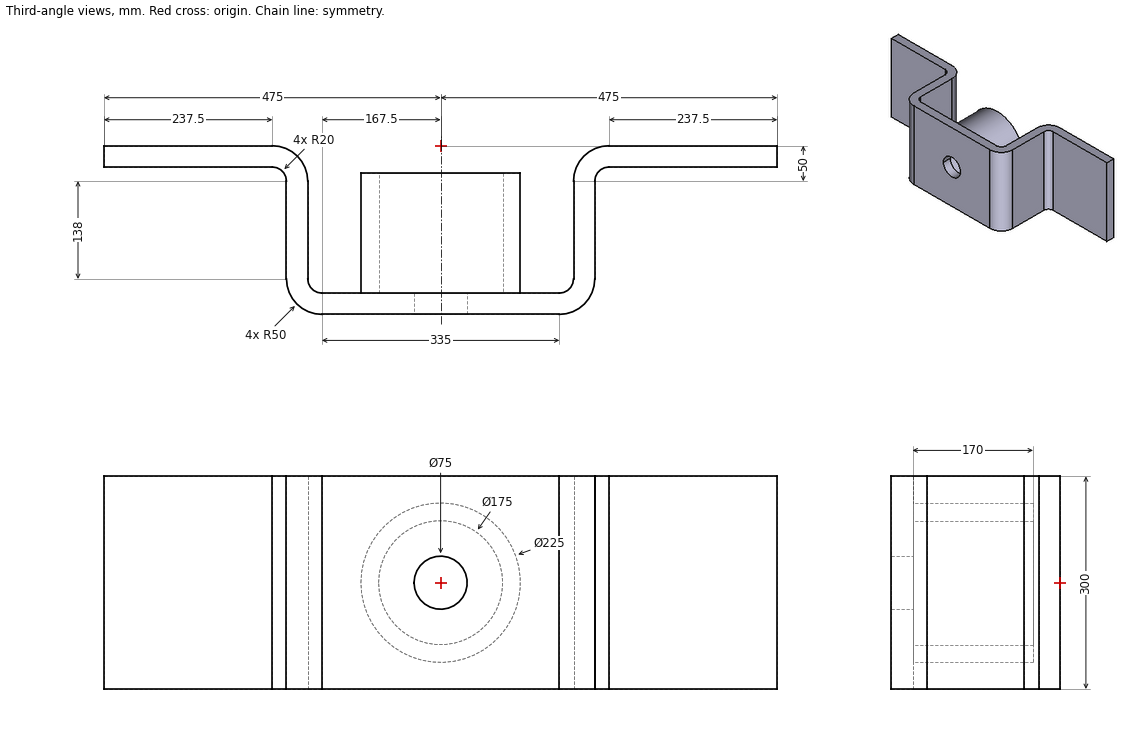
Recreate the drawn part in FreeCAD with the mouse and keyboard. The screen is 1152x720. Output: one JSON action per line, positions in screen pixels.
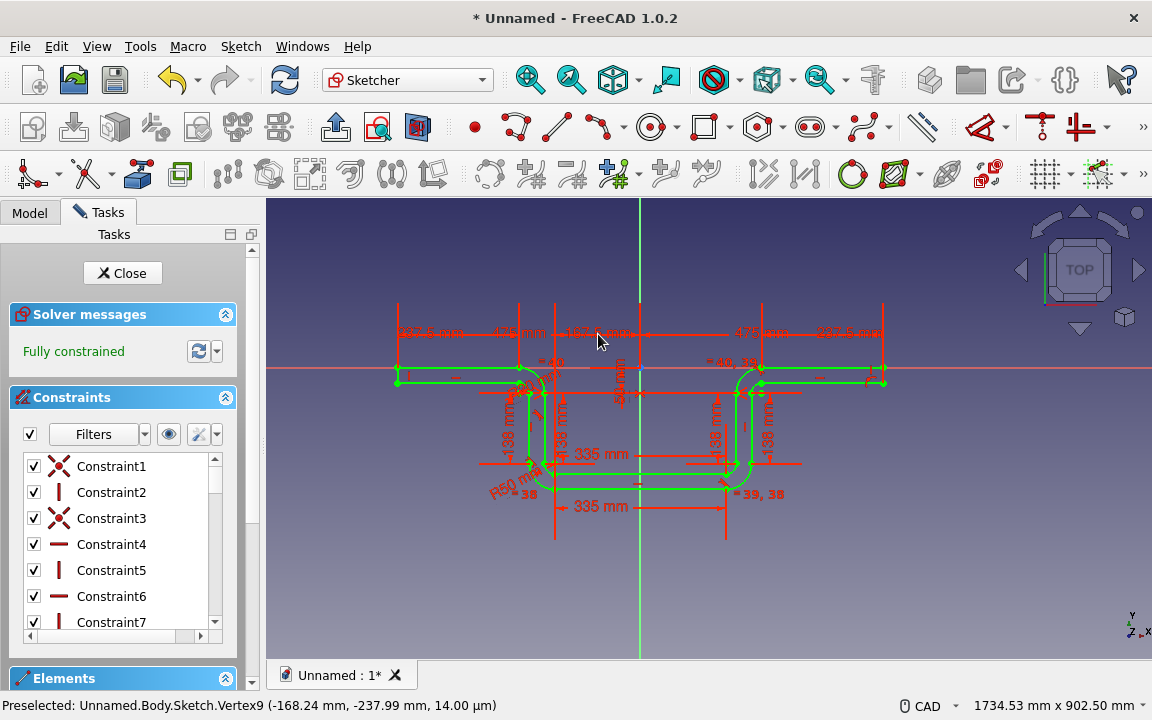
{"action": "left_click", "coordinate": [123, 273]}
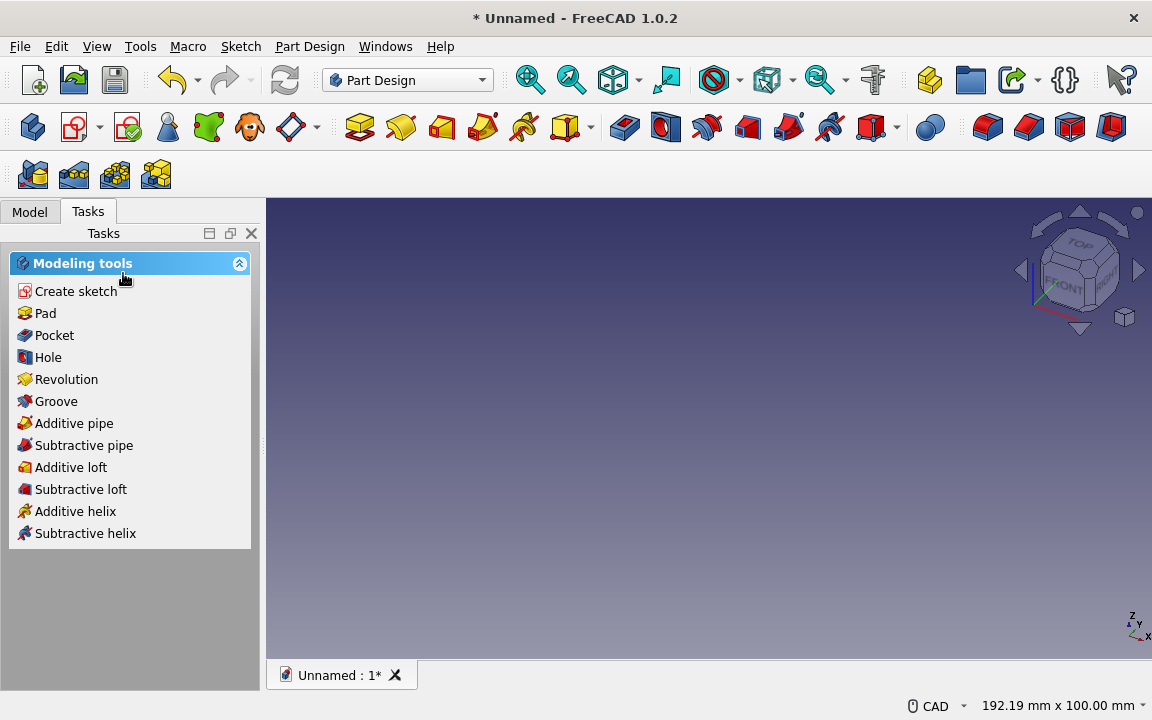
{"action": "left_click", "coordinate": [360, 128]}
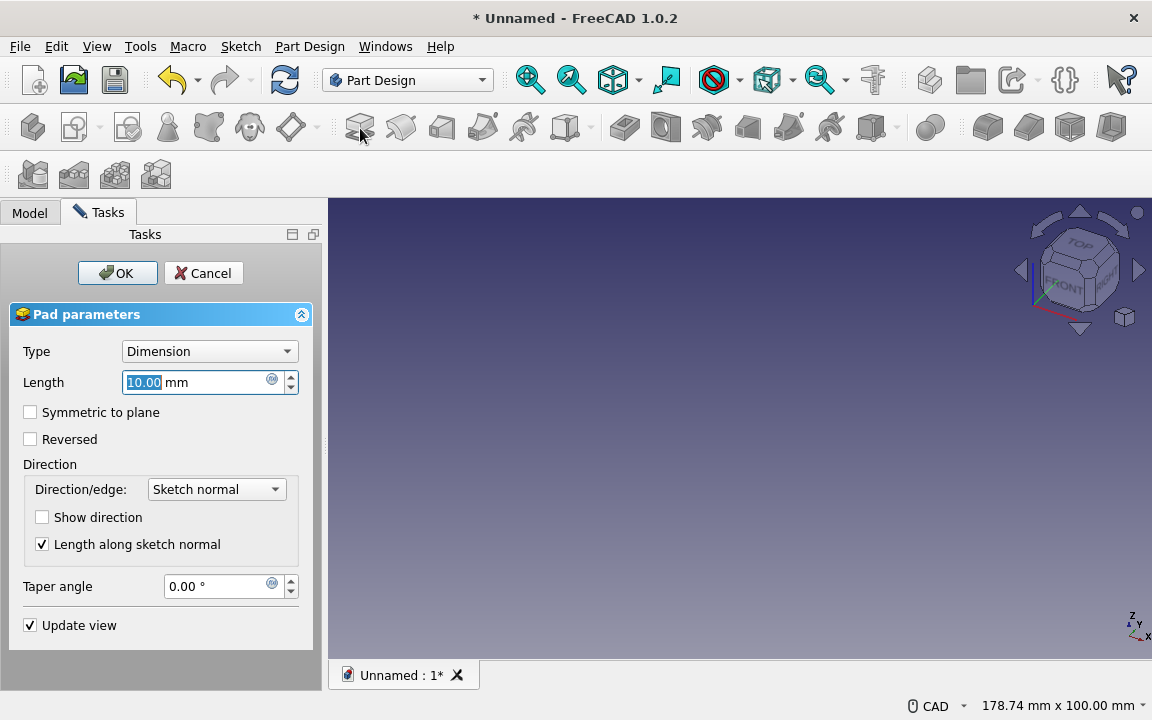
{"action": "type", "text": "300"}
{"action": "key", "text": "Tab"}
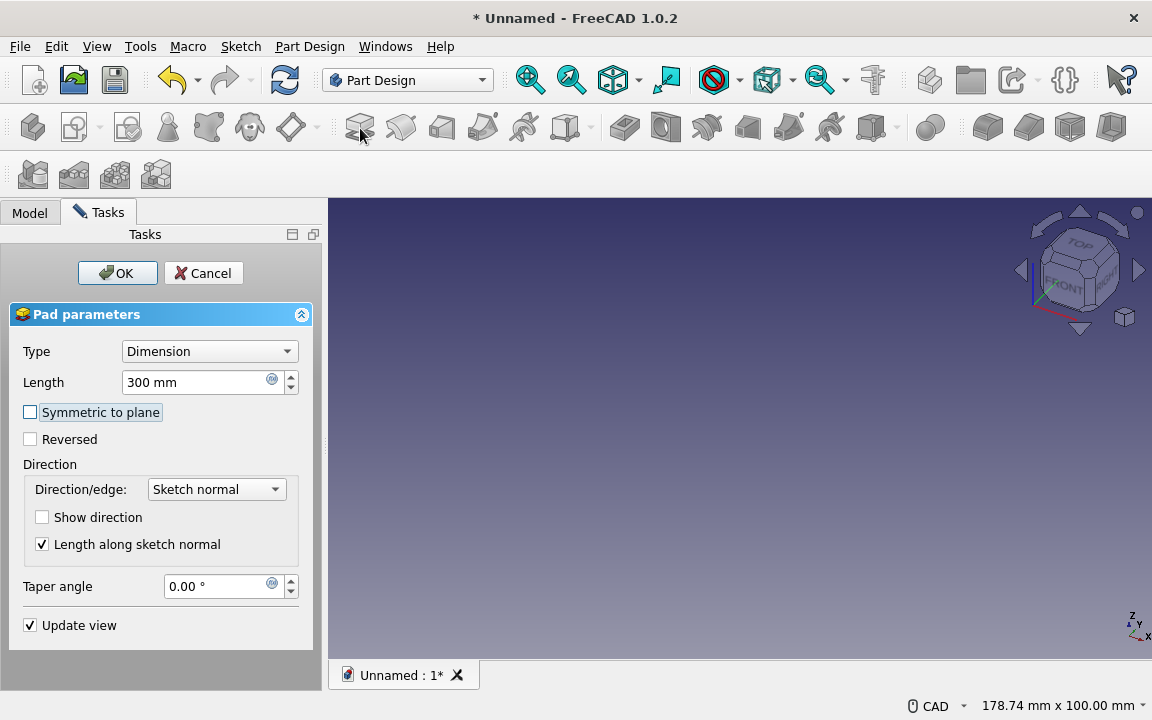
{"action": "left_click", "coordinate": [31, 412]}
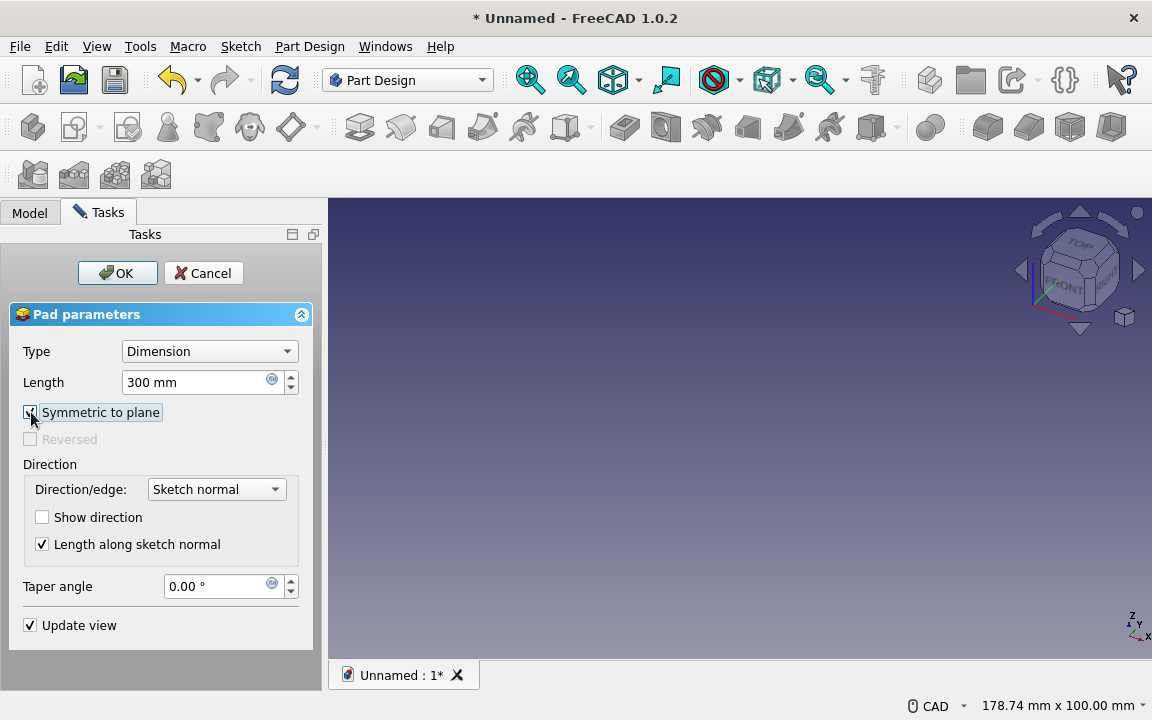
{"action": "left_click", "coordinate": [118, 273]}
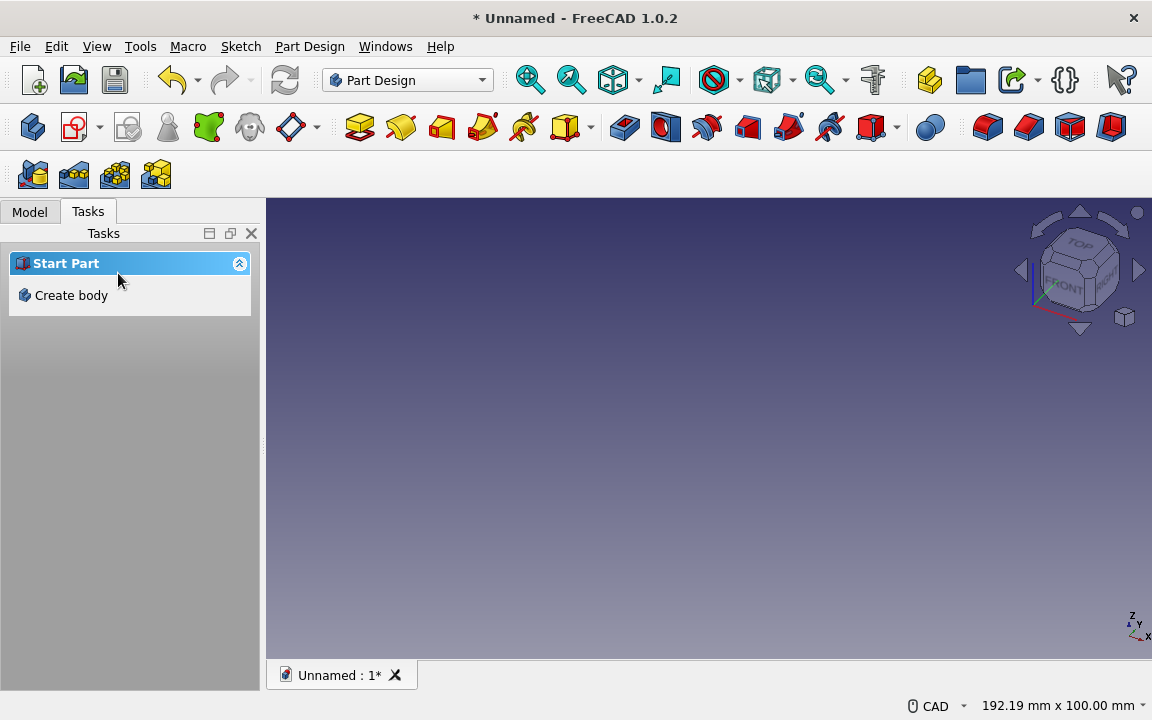
{"action": "key", "text": "v f"}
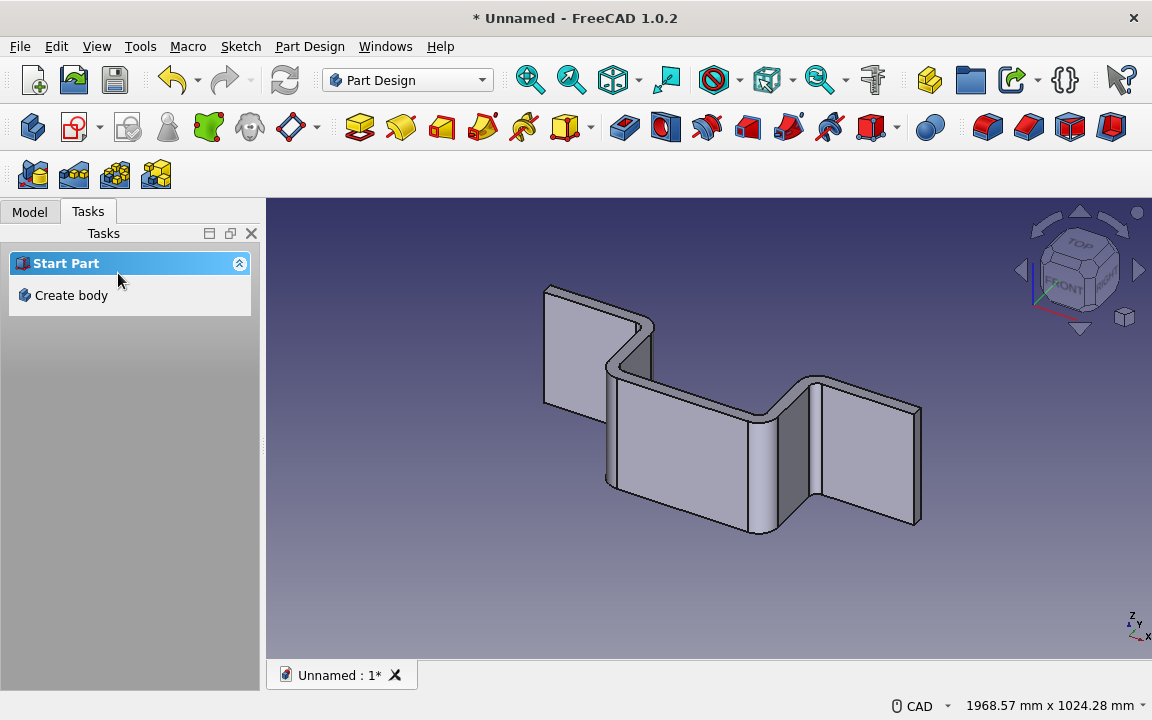
{"action": "key", "text": "4"}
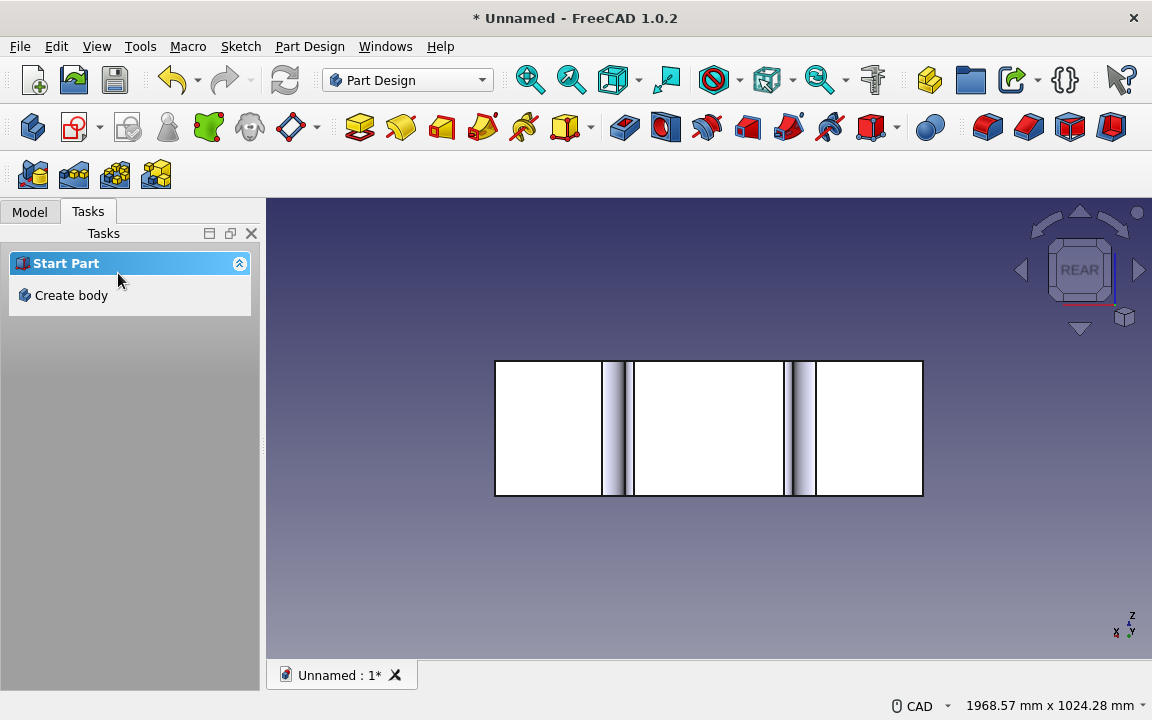
{"action": "left_click", "coordinate": [709, 427]}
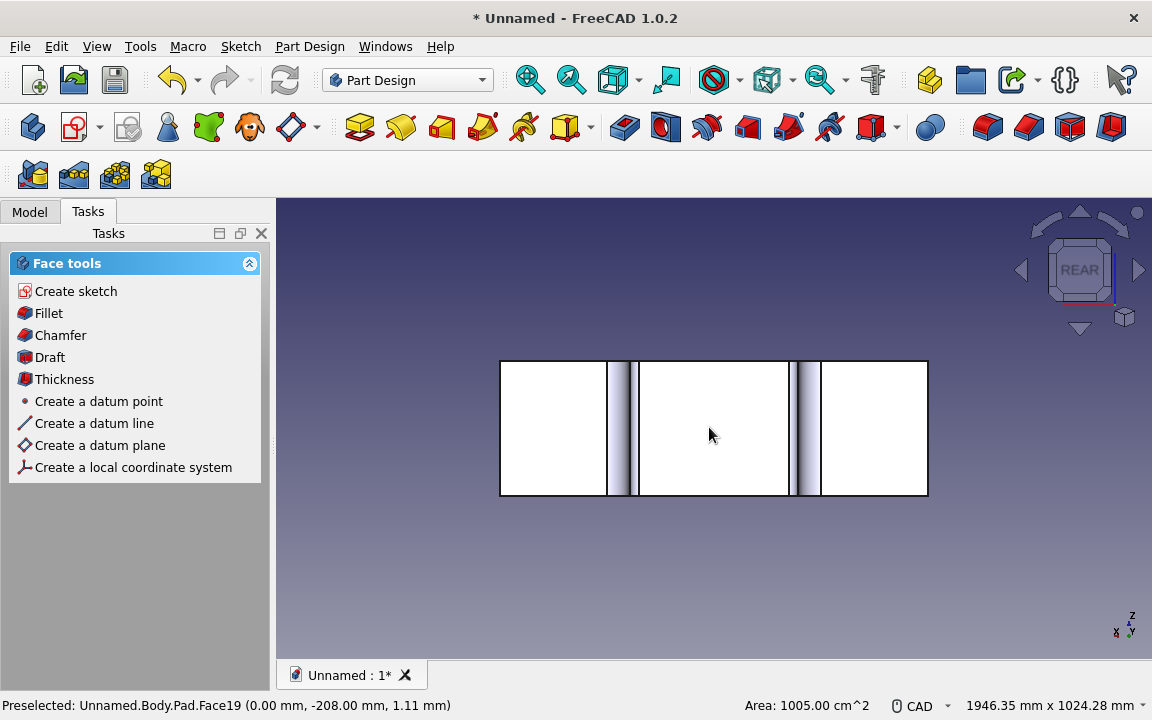
{"action": "left_click", "coordinate": [74, 128]}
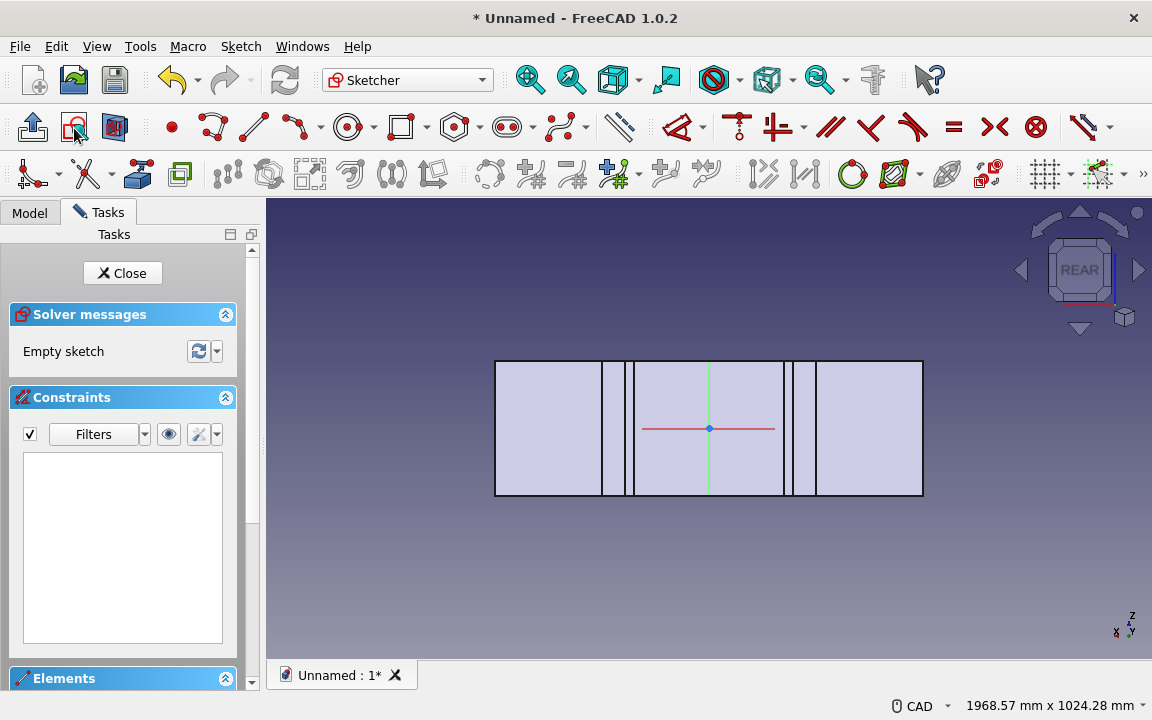
{"action": "key", "text": "q s"}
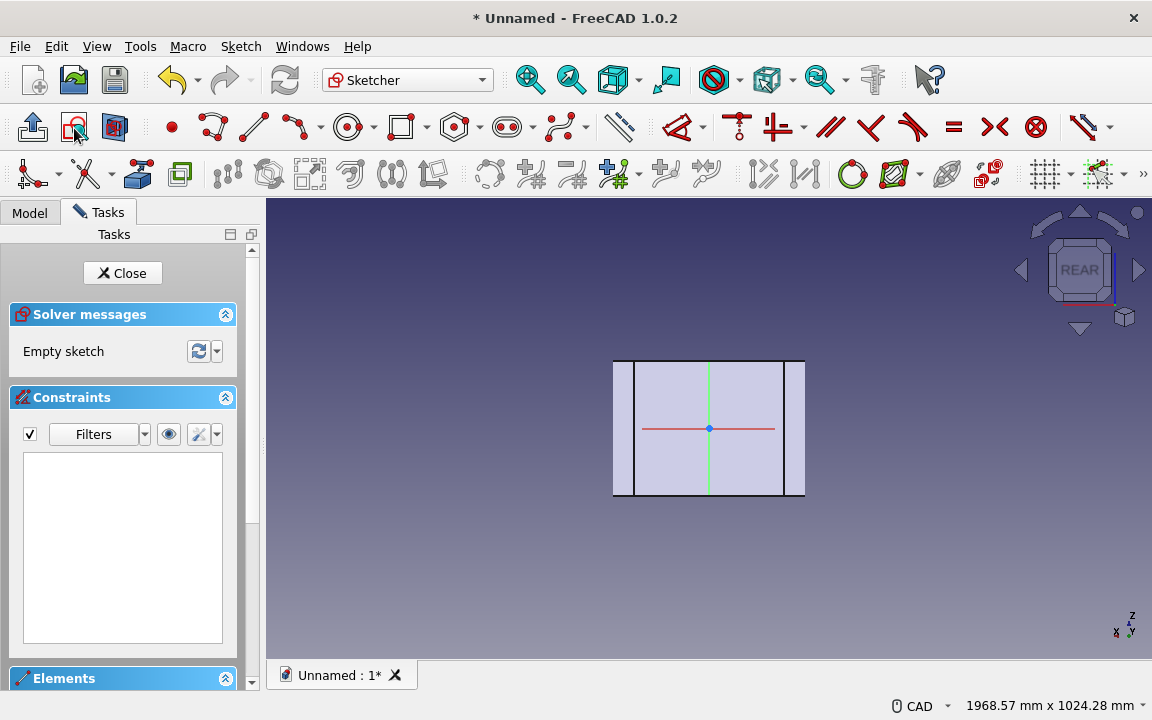
{"action": "scroll", "coordinate": [749, 428], "scroll_direction": "up", "scroll_amount": 5}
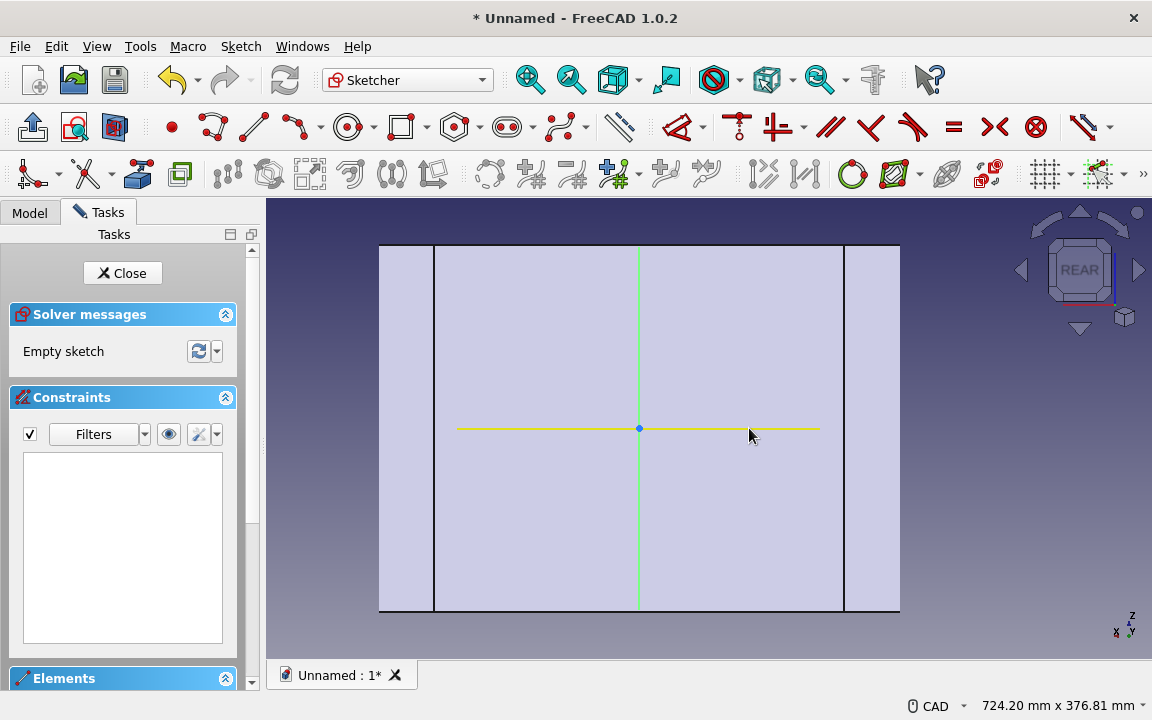
{"action": "key", "text": "g c"}